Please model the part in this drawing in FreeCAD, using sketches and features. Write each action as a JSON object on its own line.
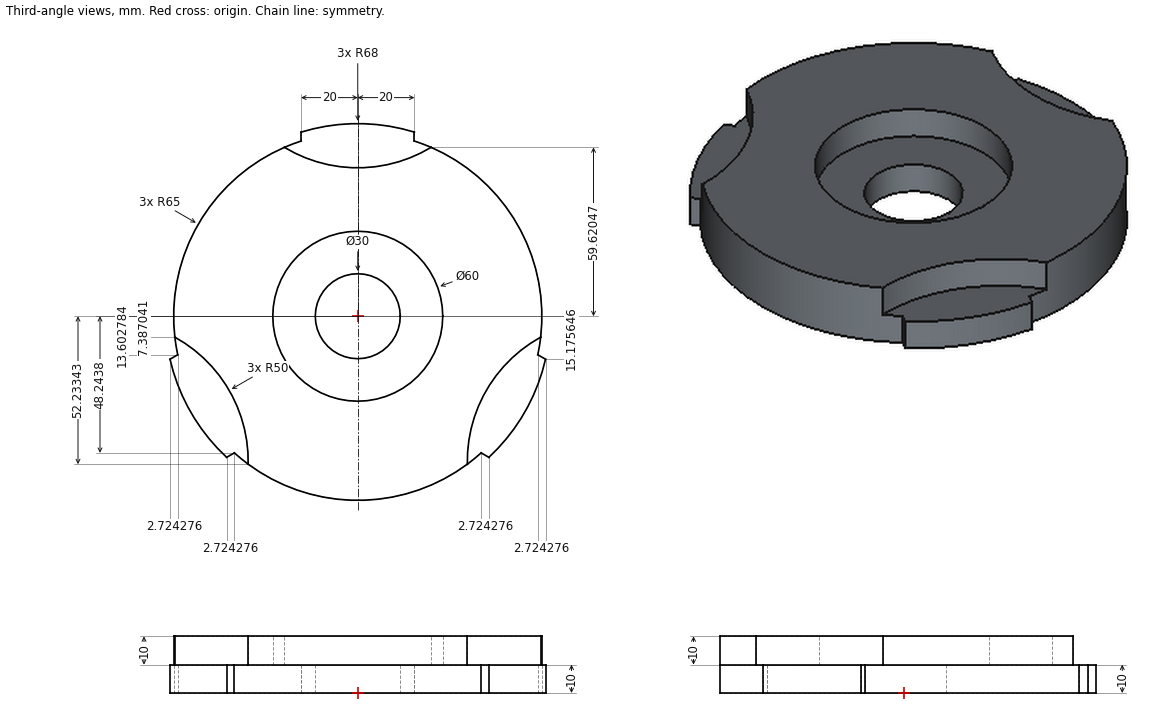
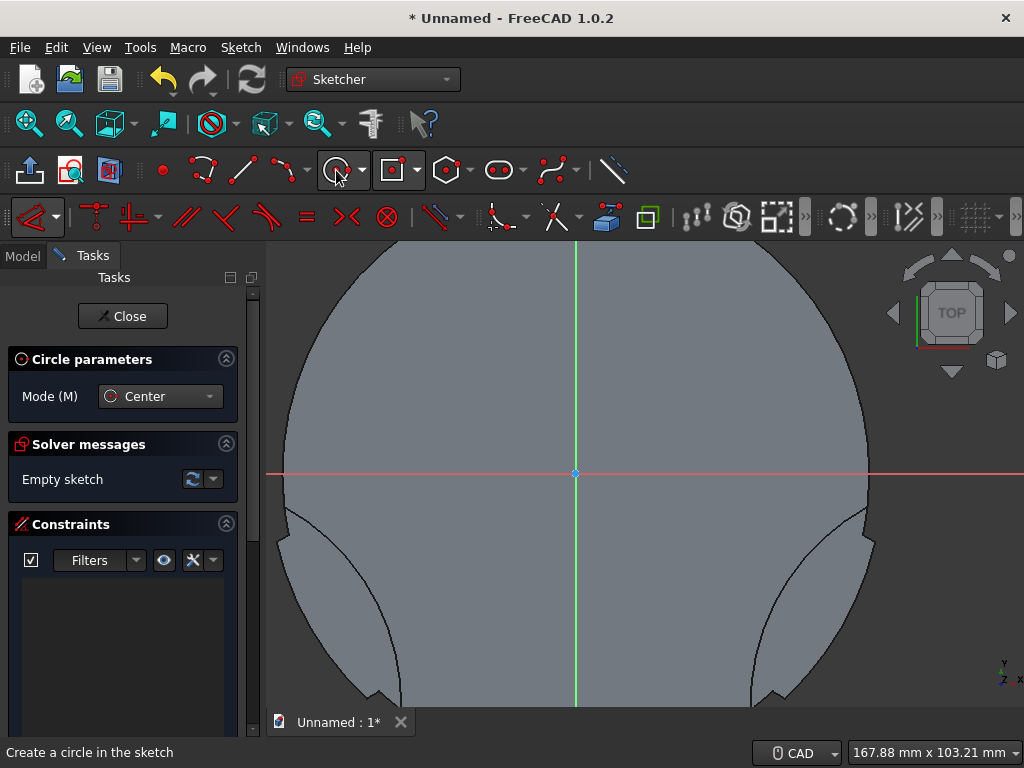
{"action": "left_click", "coordinate": [576, 474]}
{"action": "mouse_move", "coordinate": [672, 378]}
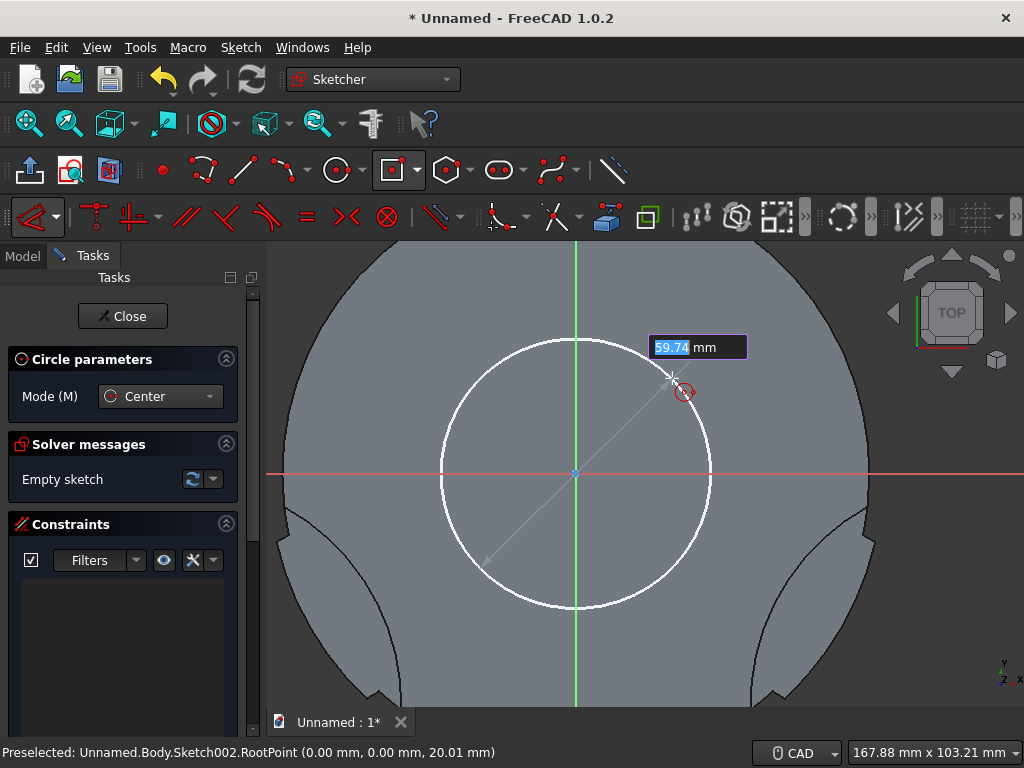
{"action": "type", "text": "60"}
{"action": "key", "text": "Return"}
{"action": "key", "text": "Escape"}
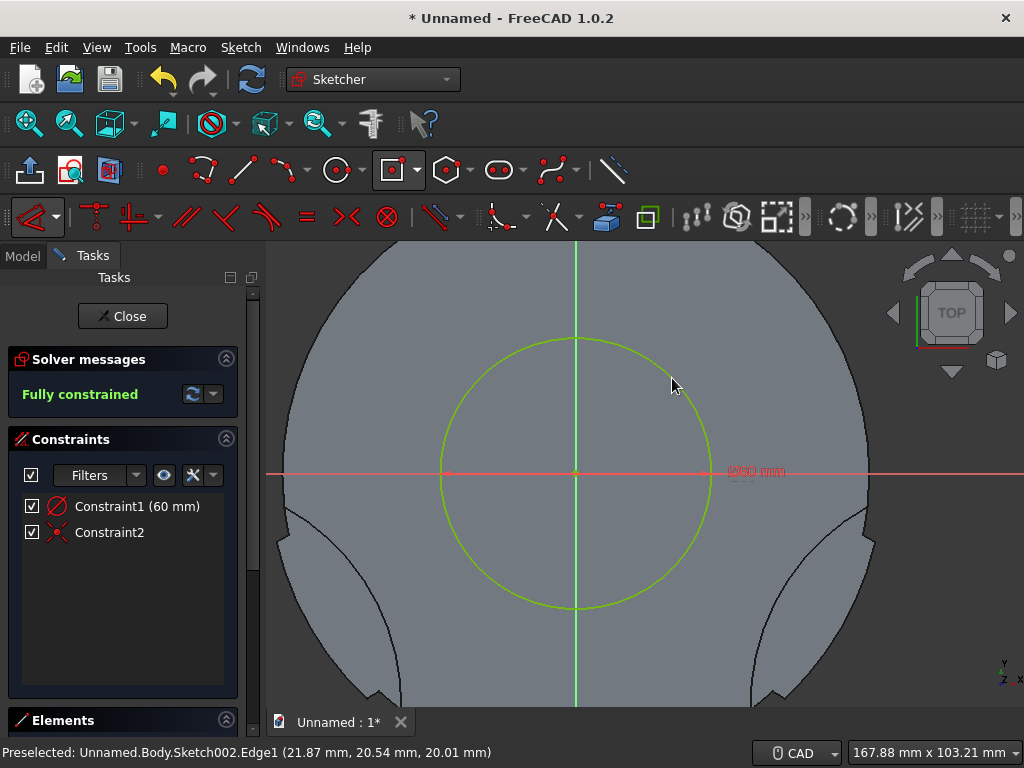
{"action": "left_click", "coordinate": [123, 316]}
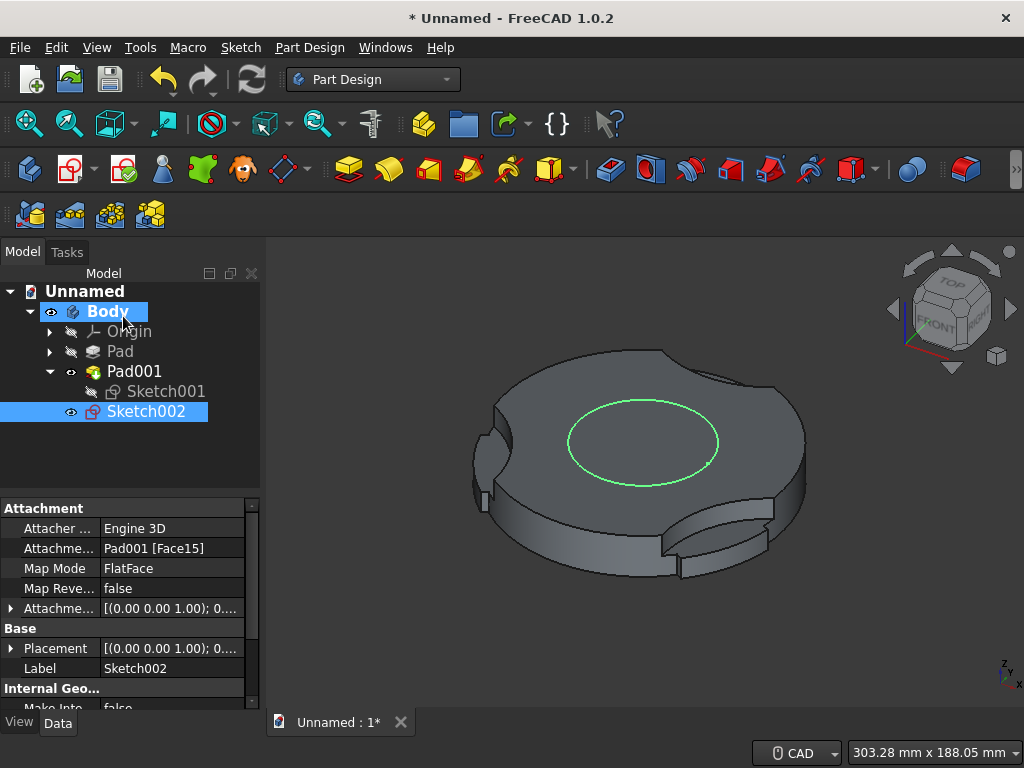
{"action": "left_click", "coordinate": [612, 170]}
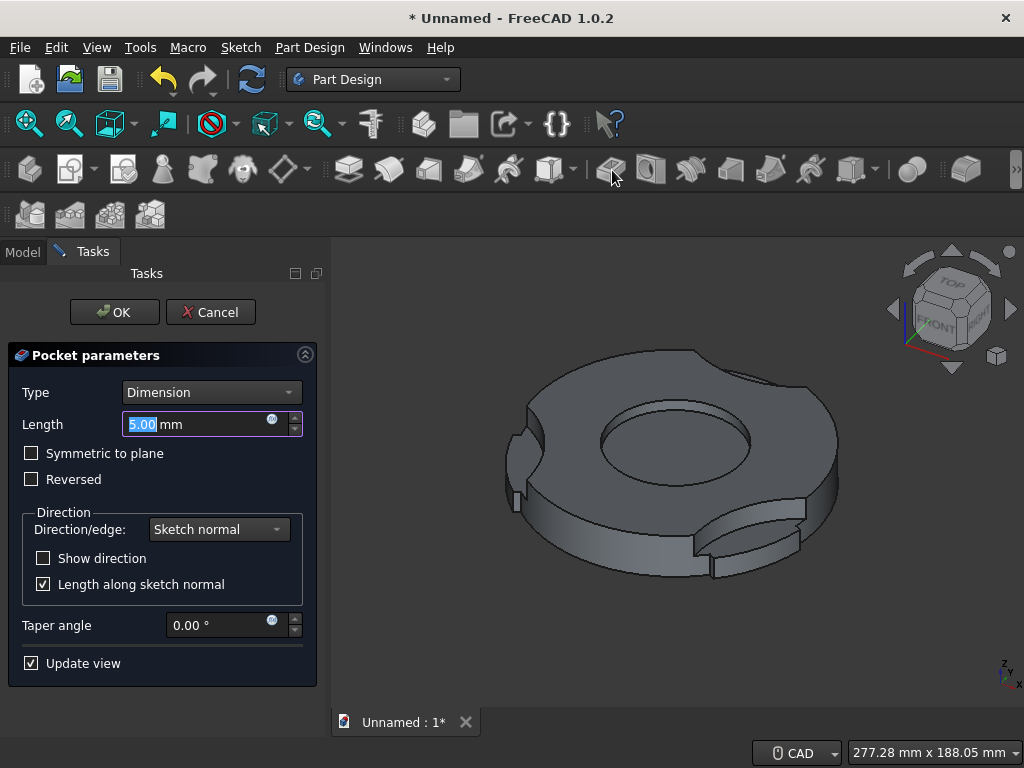
{"action": "type", "text": "10"}
{"action": "key", "text": "Tab"}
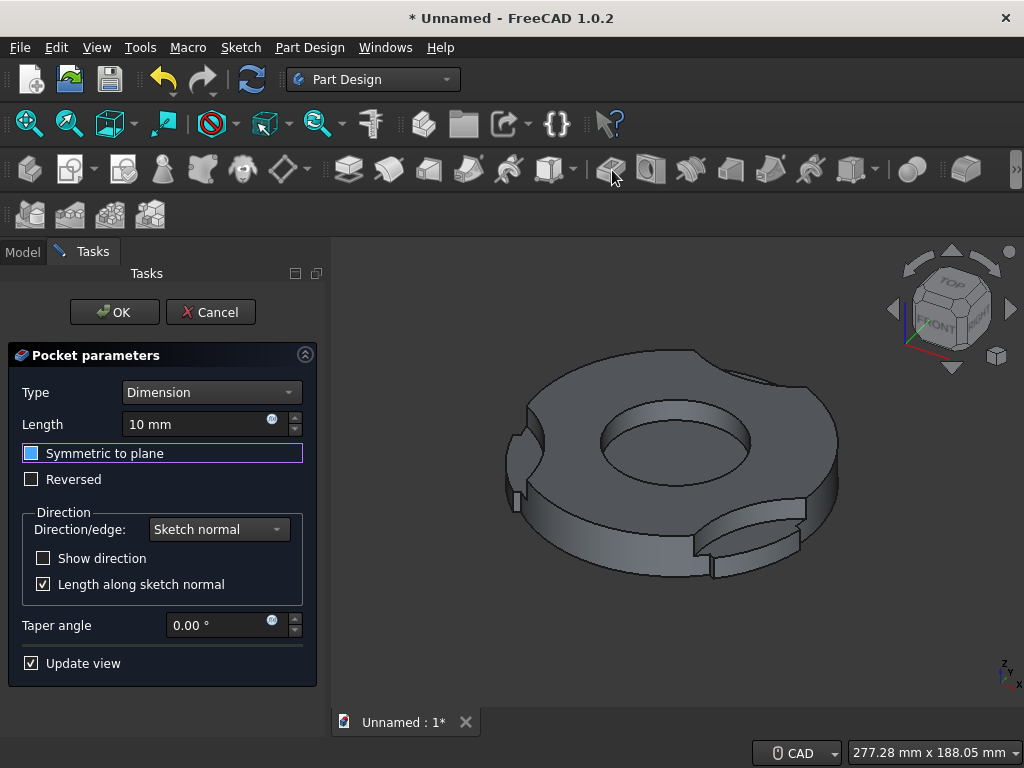
{"action": "left_click", "coordinate": [115, 312]}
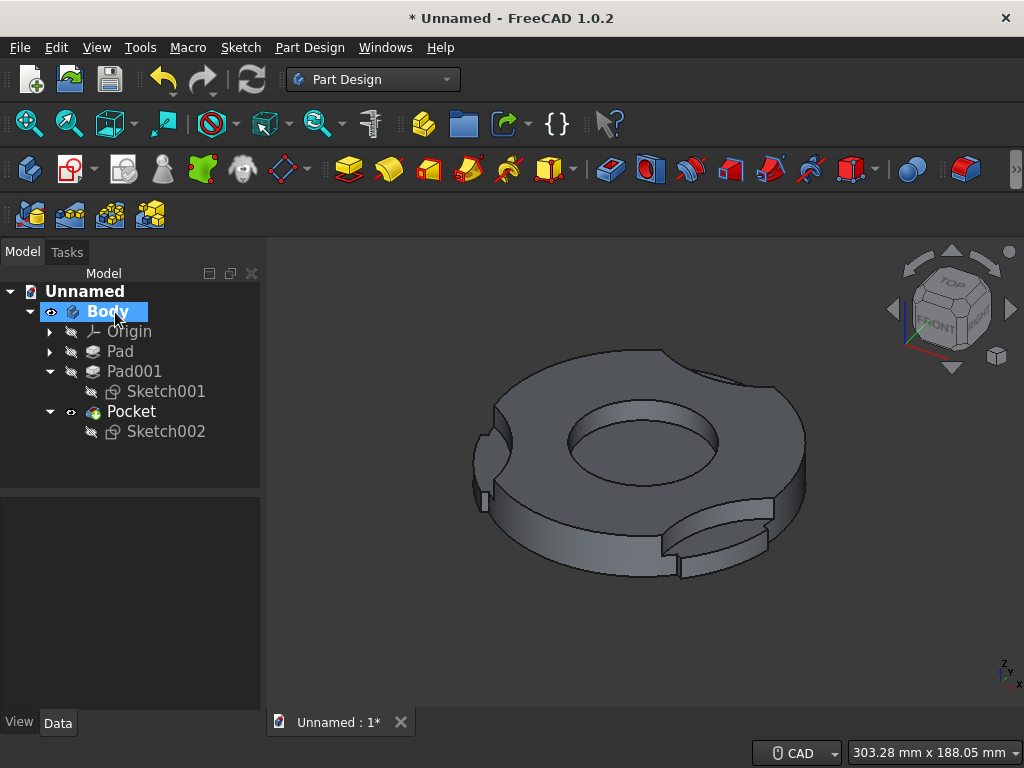
{"action": "left_click", "coordinate": [643, 462]}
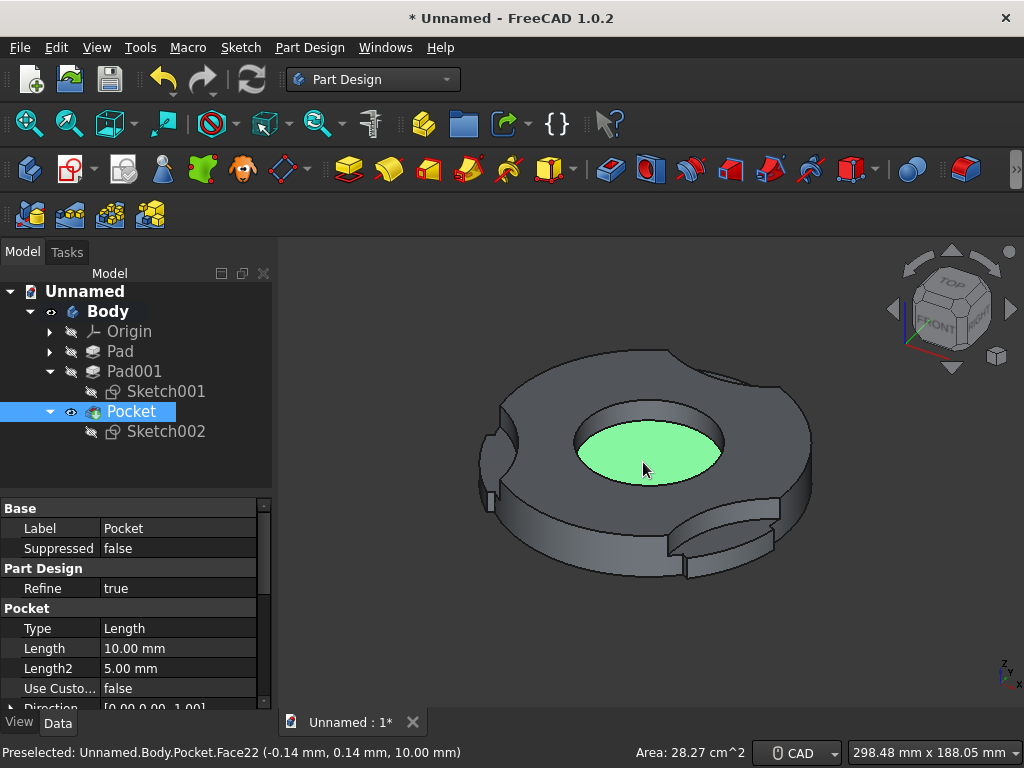
{"action": "left_click", "coordinate": [70, 170]}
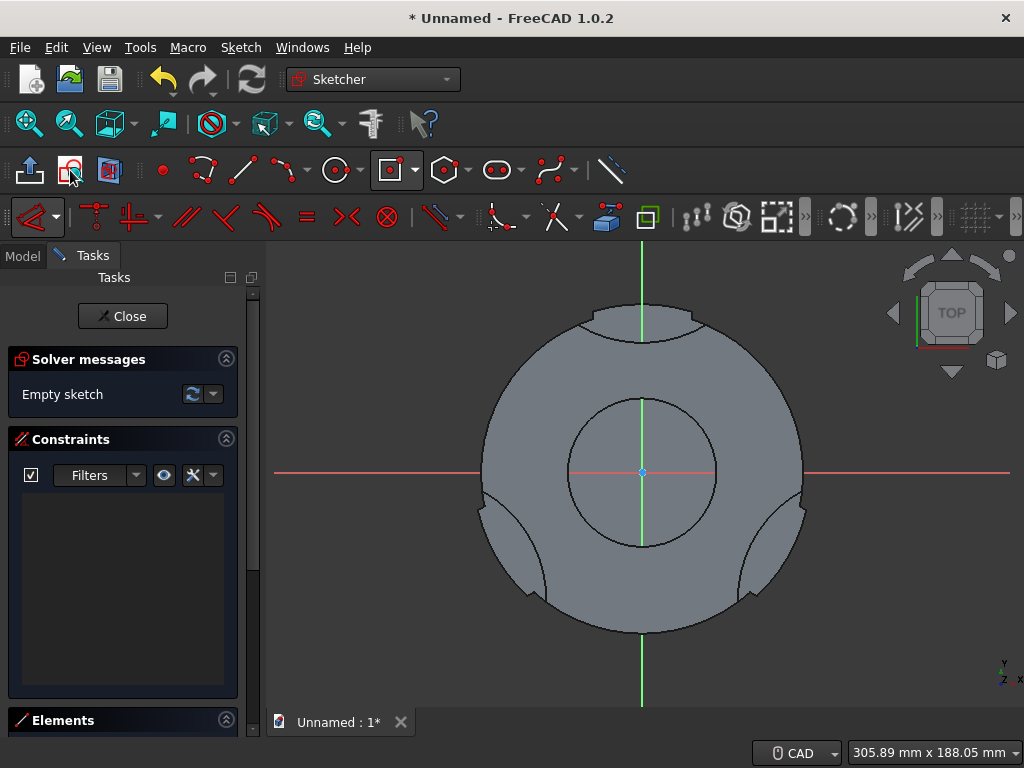
{"action": "scroll", "coordinate": [664, 472], "scroll_direction": "up", "scroll_amount": 7}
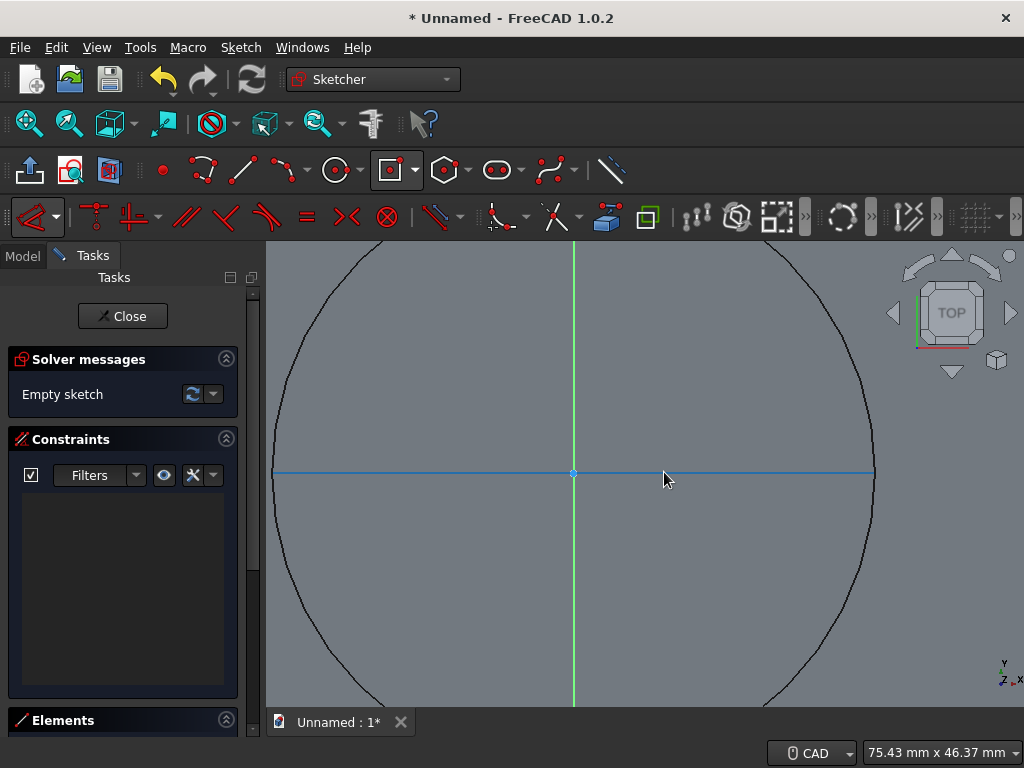
{"action": "left_click", "coordinate": [336, 170]}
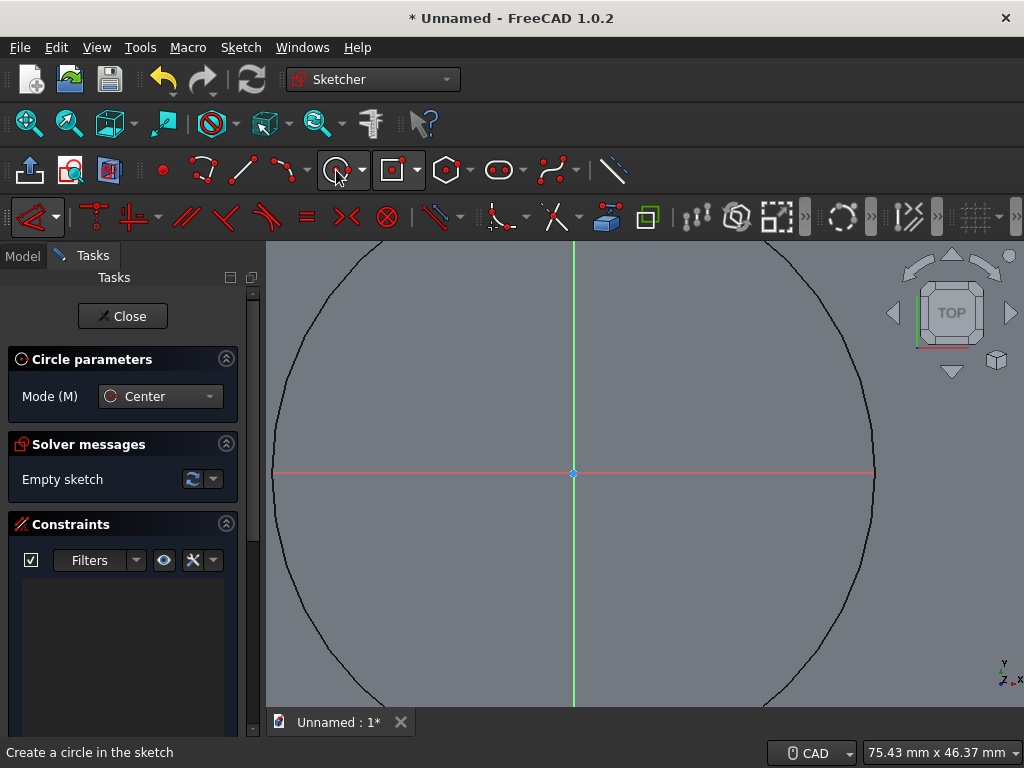
{"action": "left_click", "coordinate": [574, 473]}
{"action": "mouse_move", "coordinate": [680, 367]}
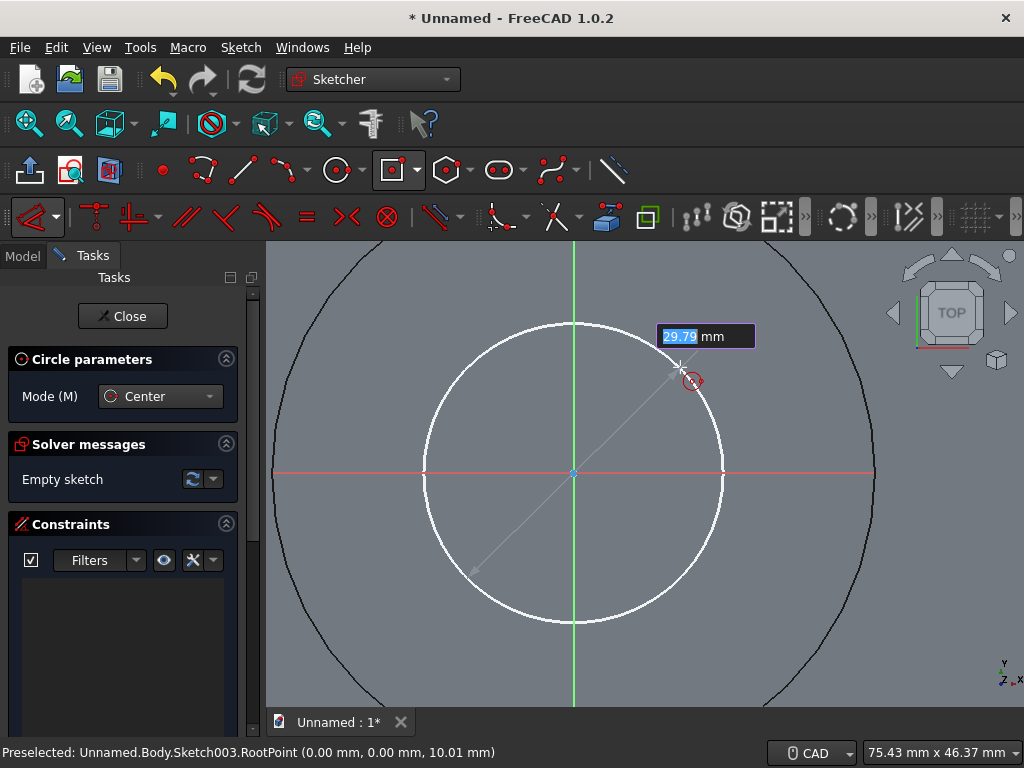
{"action": "type", "text": "30"}
{"action": "key", "text": "Return"}
{"action": "key", "text": "Escape"}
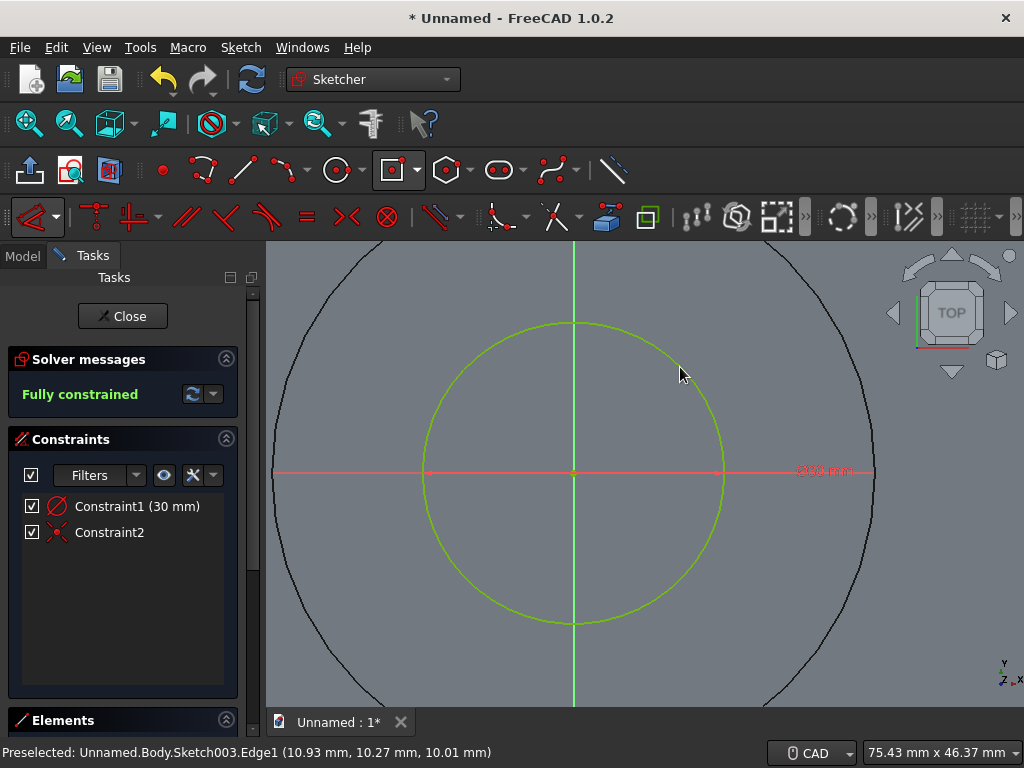
{"action": "left_click", "coordinate": [123, 316]}